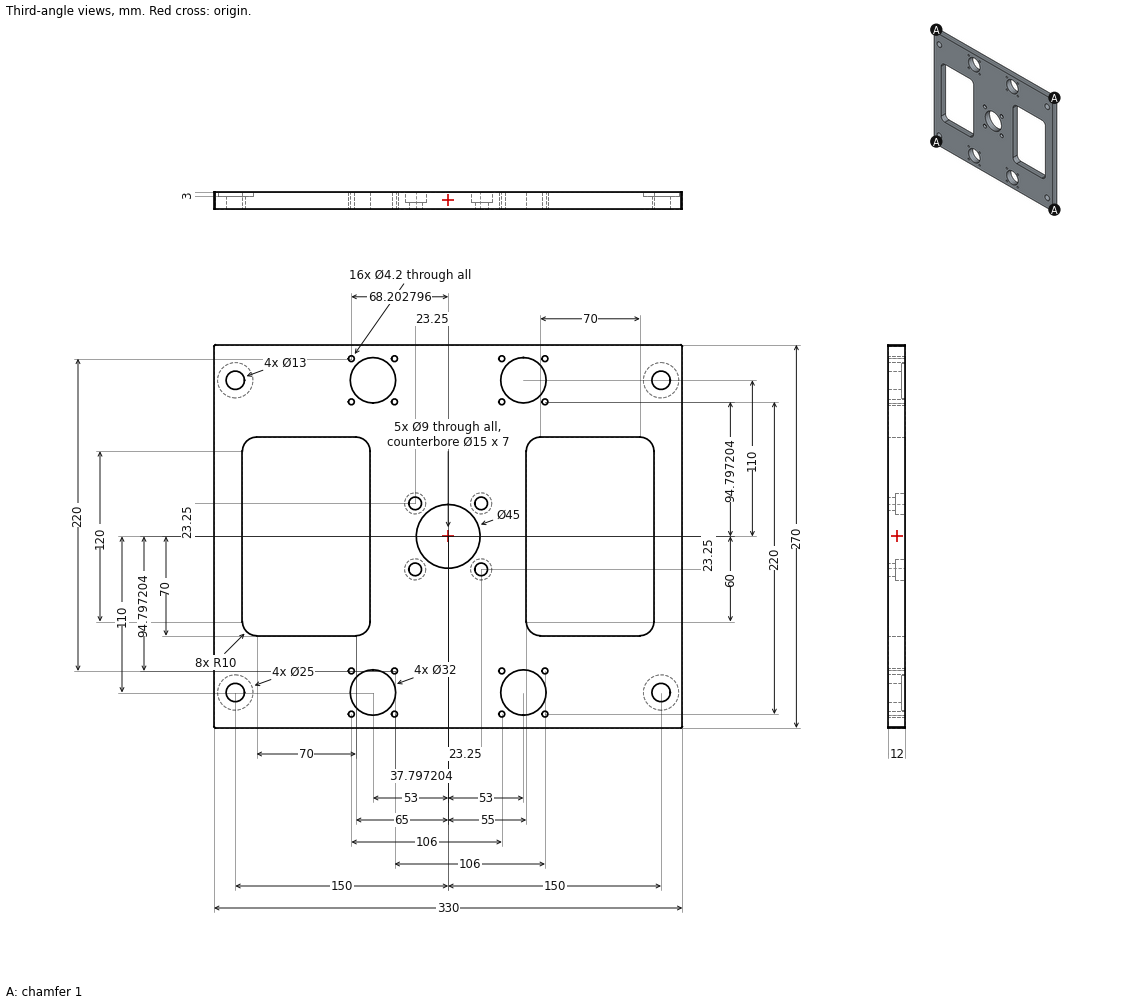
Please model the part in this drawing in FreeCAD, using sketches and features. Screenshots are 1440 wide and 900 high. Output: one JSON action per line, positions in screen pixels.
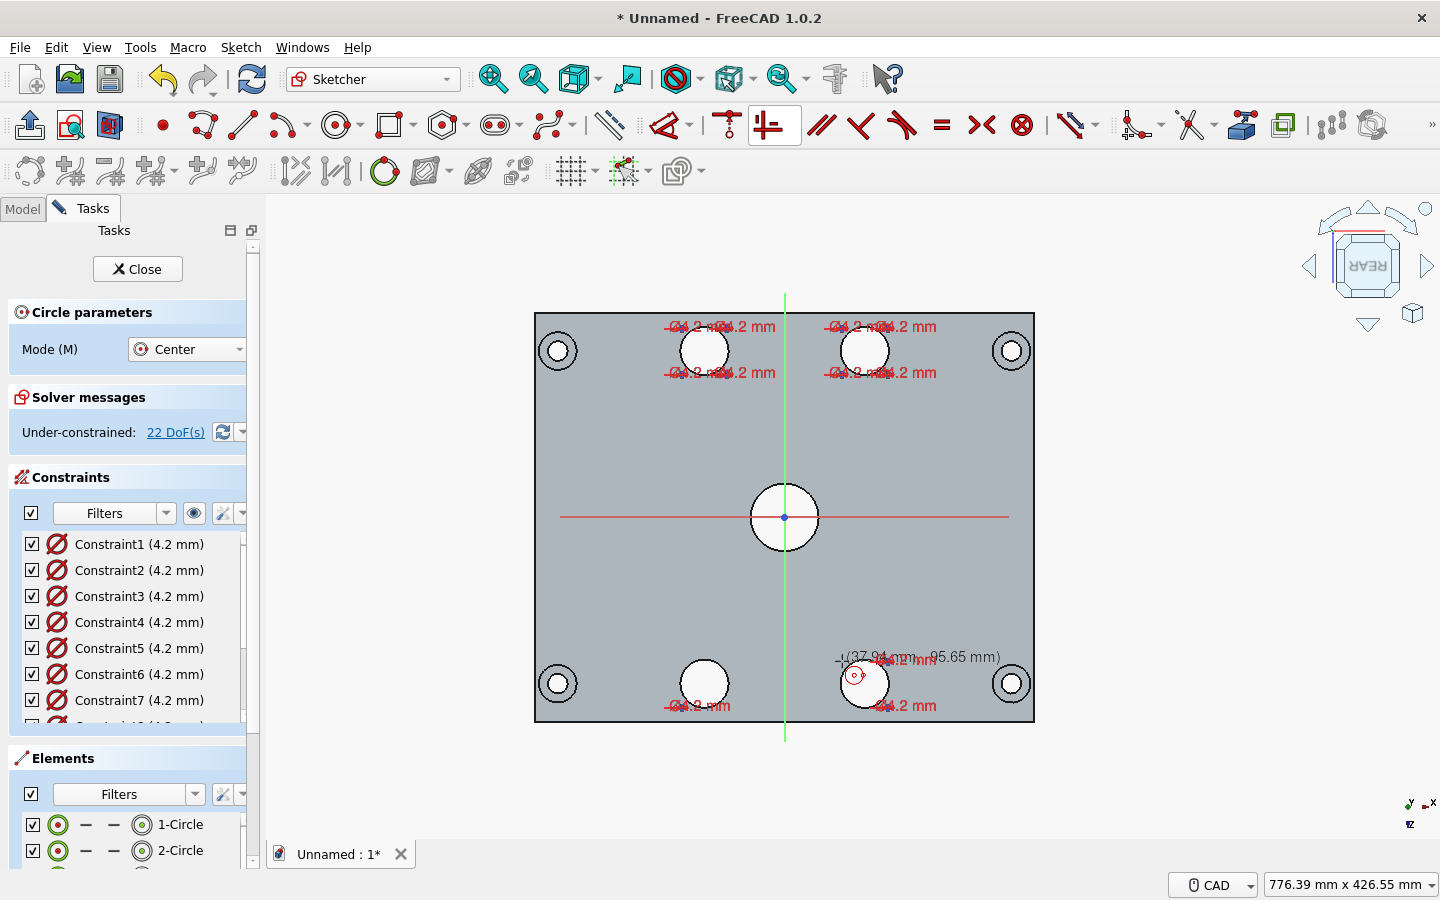
{"action": "left_click", "coordinate": [842, 661]}
{"action": "mouse_move", "coordinate": [844, 658]}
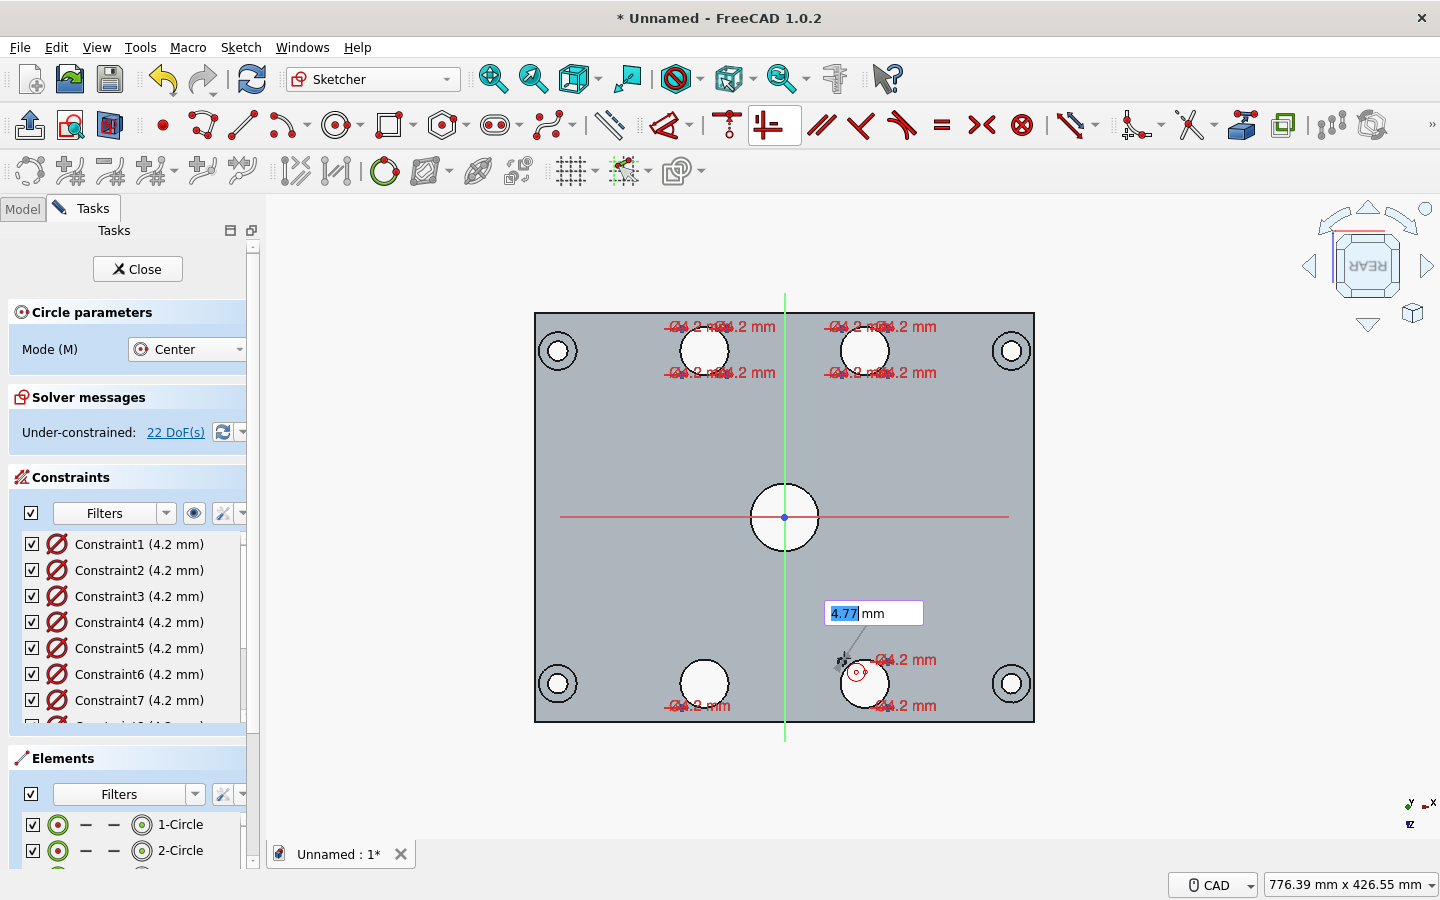
{"action": "type", "text": "4.2"}
{"action": "key", "text": "Return"}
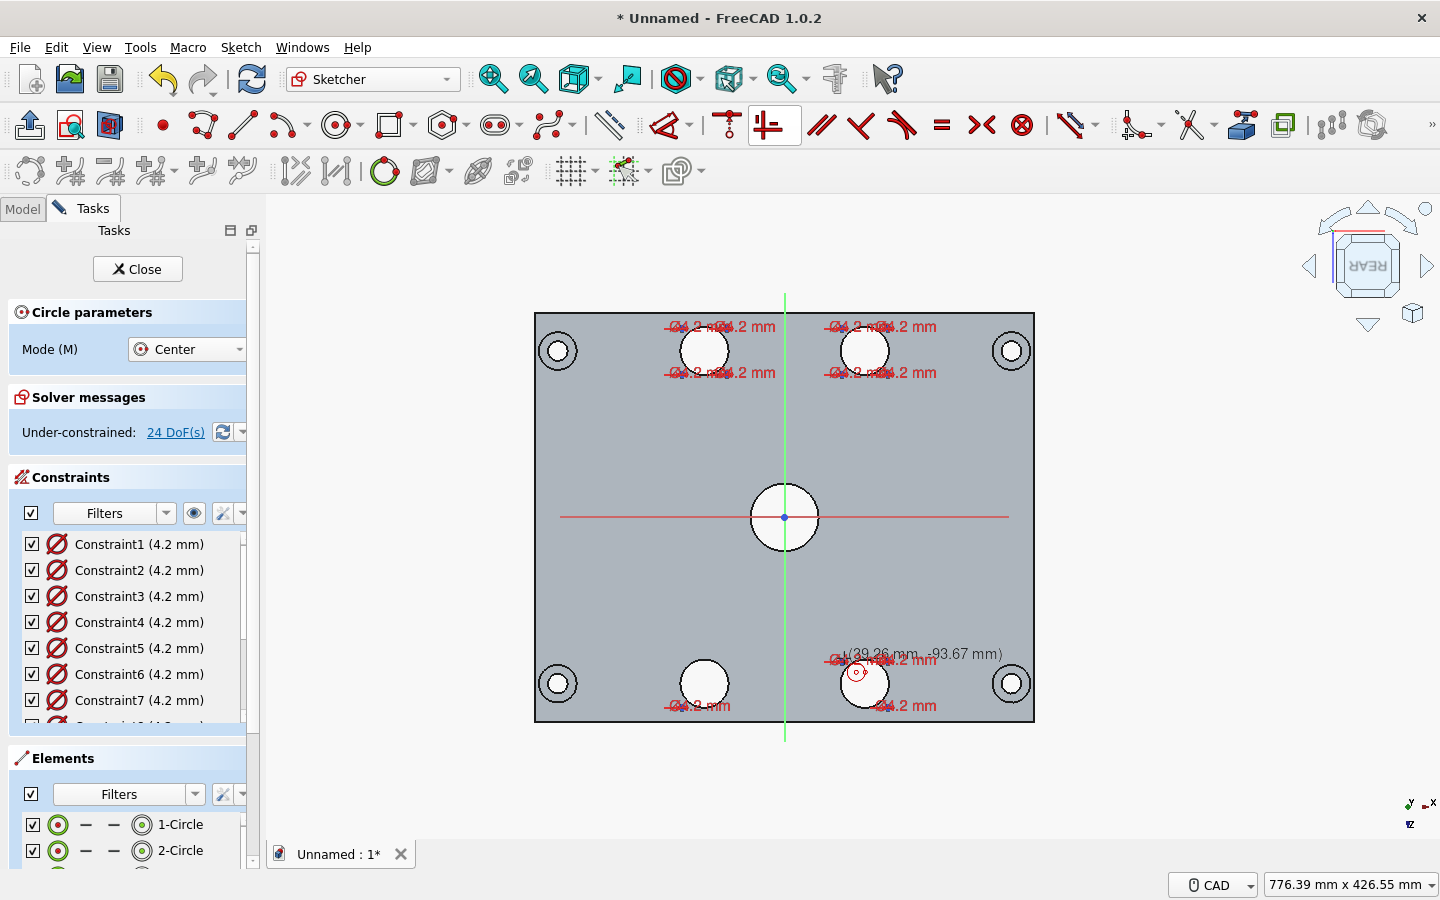
{"action": "scroll", "coordinate": [842, 707], "scroll_direction": "up", "scroll_amount": 10}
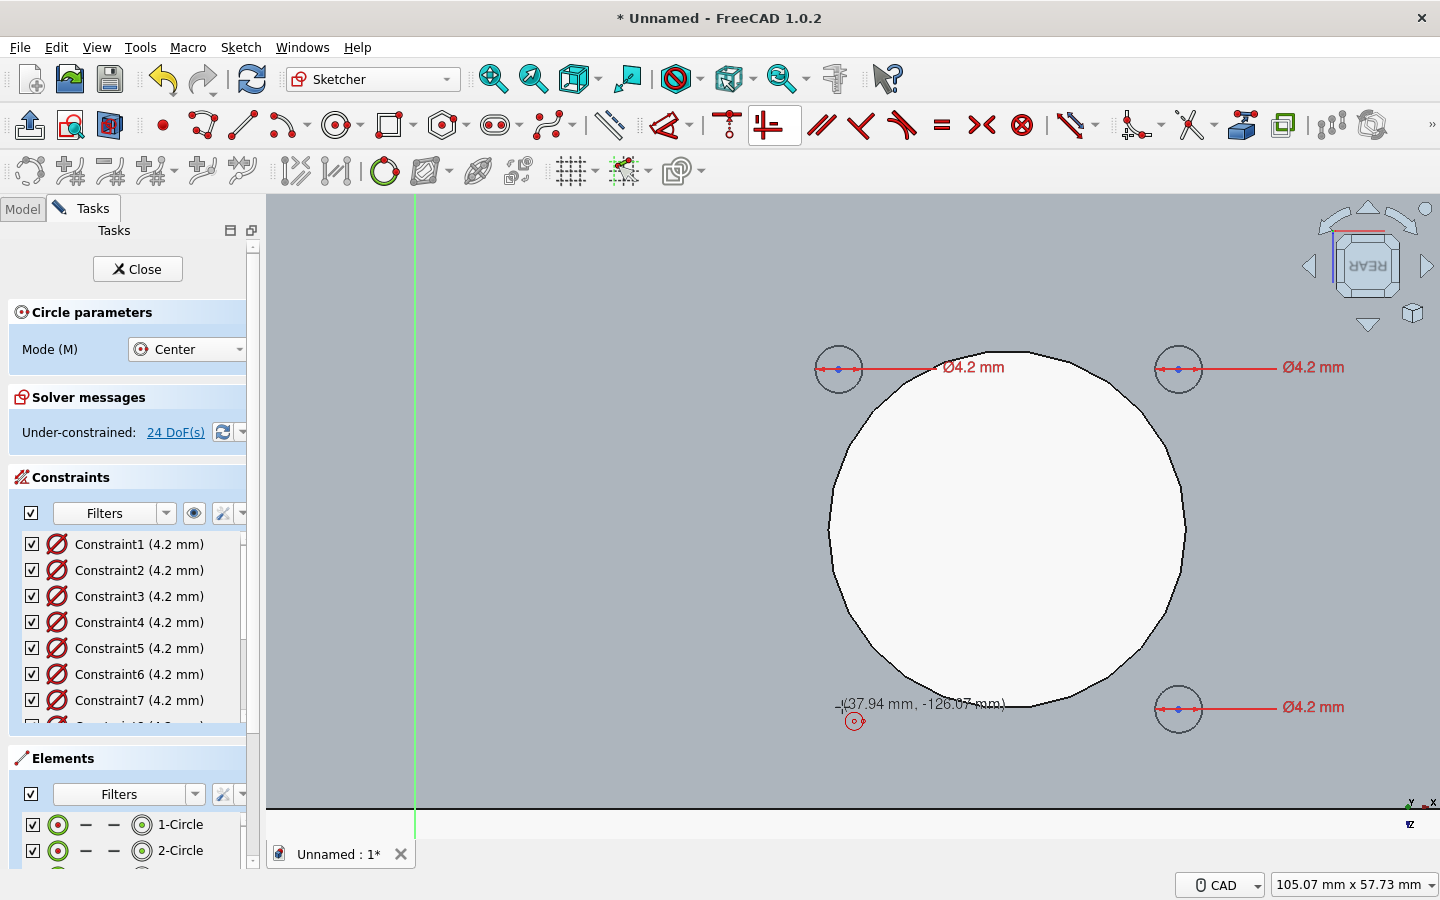
{"action": "scroll", "coordinate": [842, 707], "scroll_direction": "down", "scroll_amount": 10}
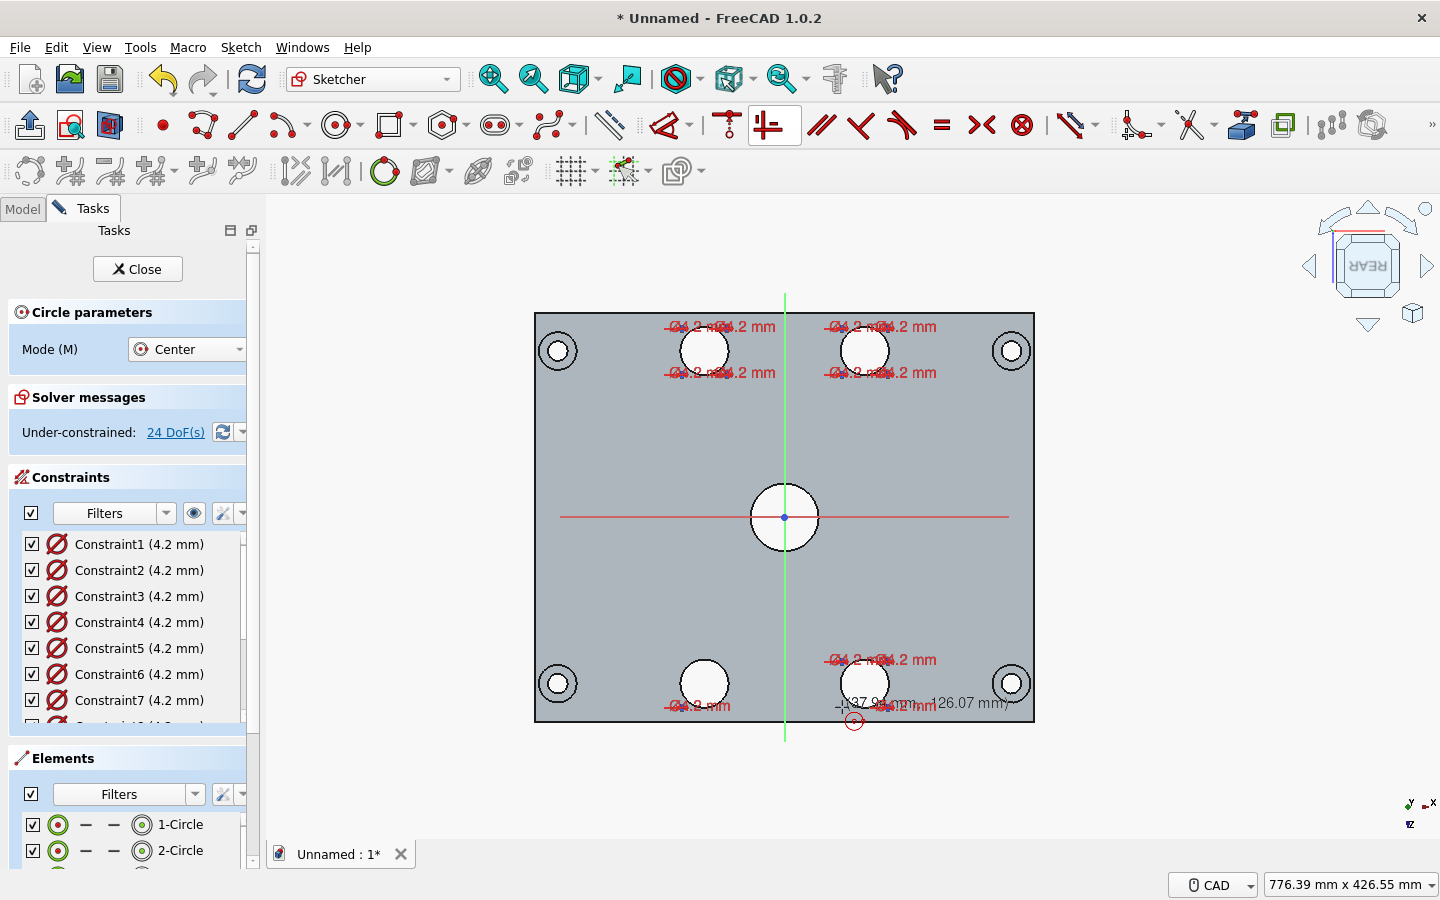
{"action": "left_click", "coordinate": [842, 707]}
{"action": "mouse_move", "coordinate": [844, 704]}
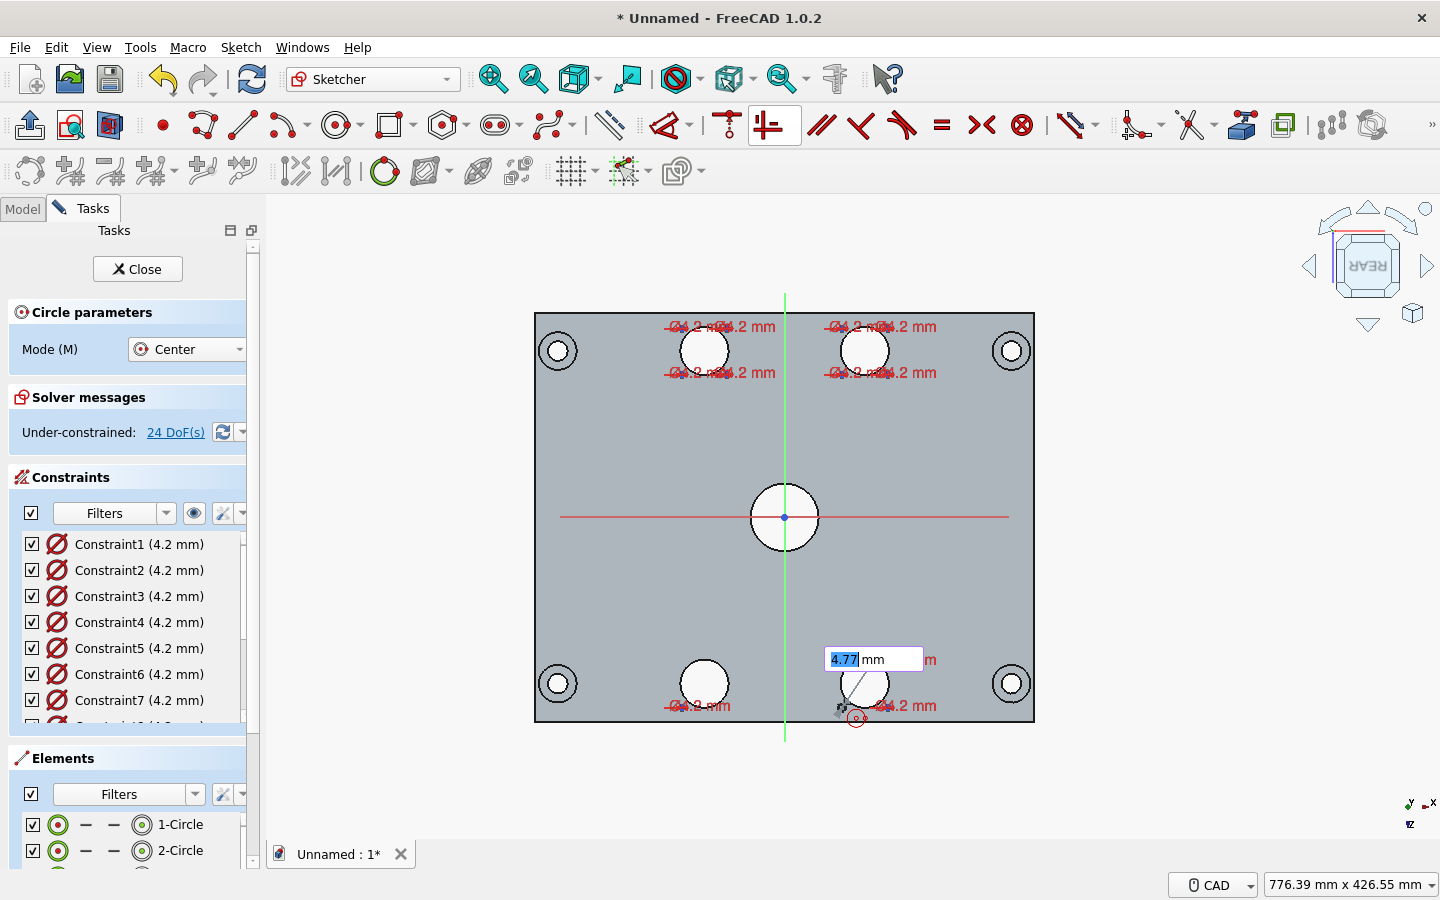
{"action": "type", "text": "4.2"}
{"action": "key", "text": "Return"}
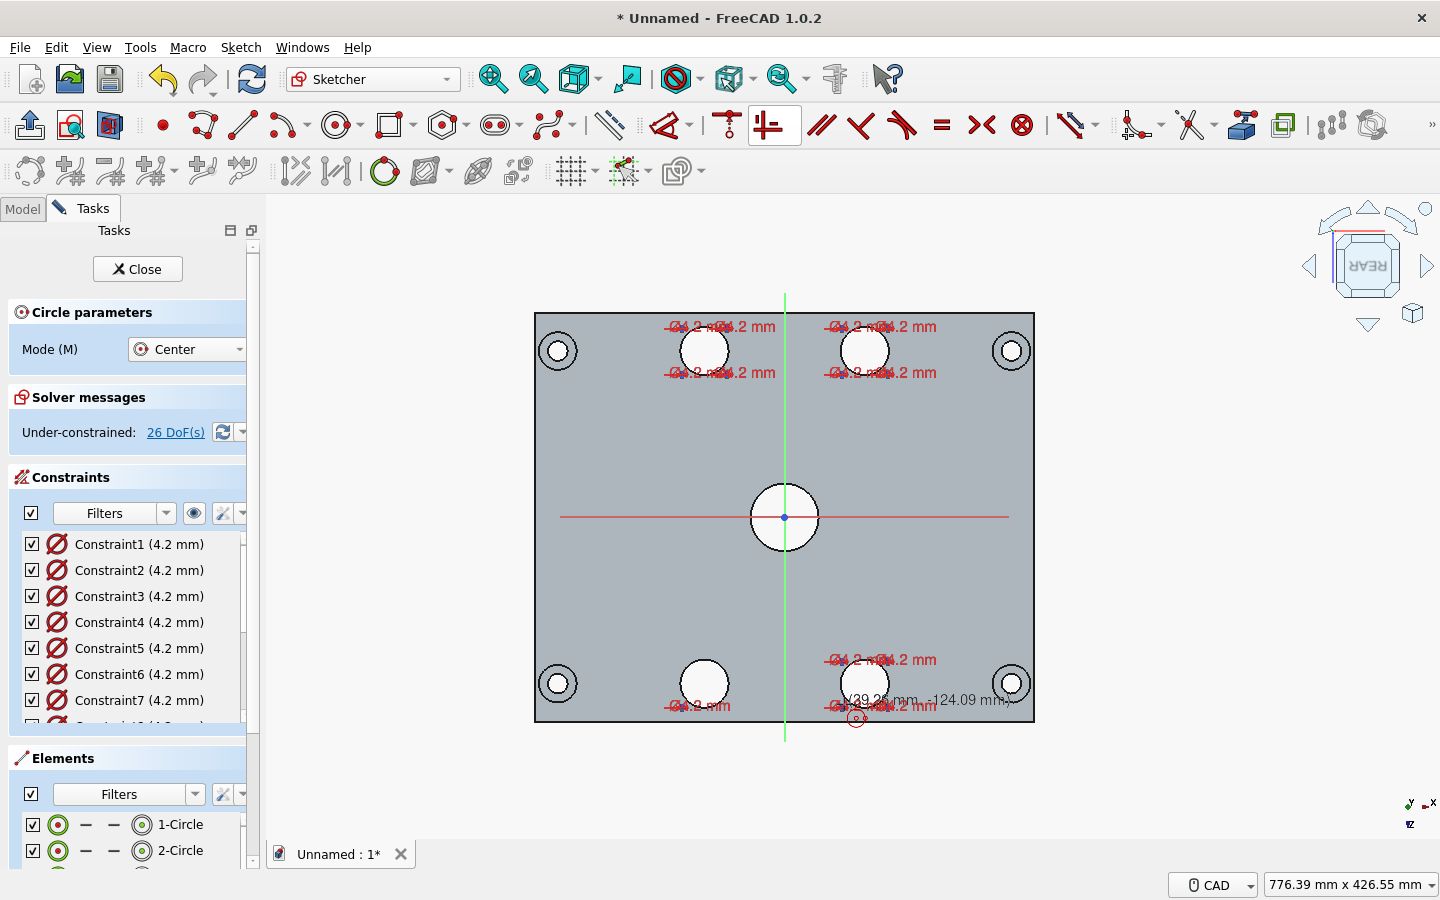
{"action": "scroll", "coordinate": [727, 707], "scroll_direction": "up", "scroll_amount": 10}